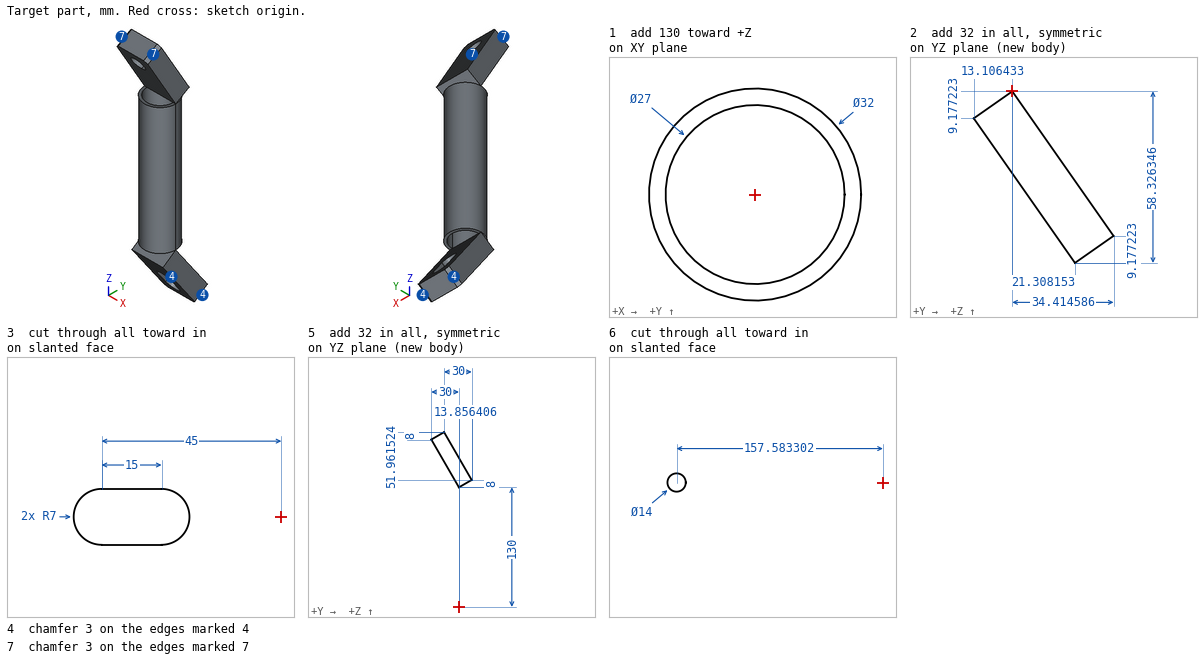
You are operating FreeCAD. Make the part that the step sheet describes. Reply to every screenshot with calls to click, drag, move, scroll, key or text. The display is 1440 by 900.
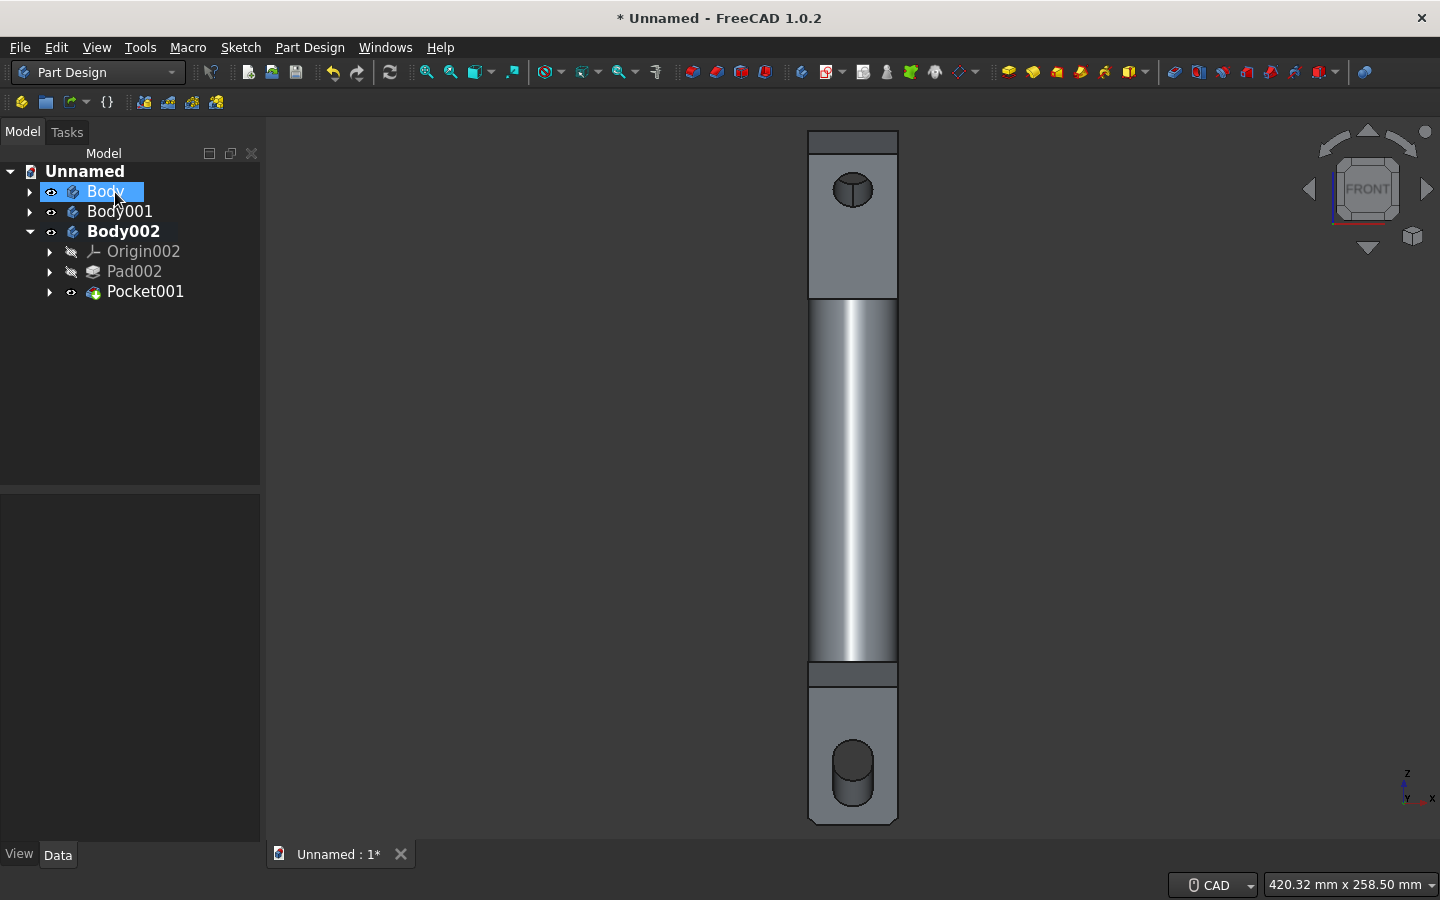
key(v)
key(f)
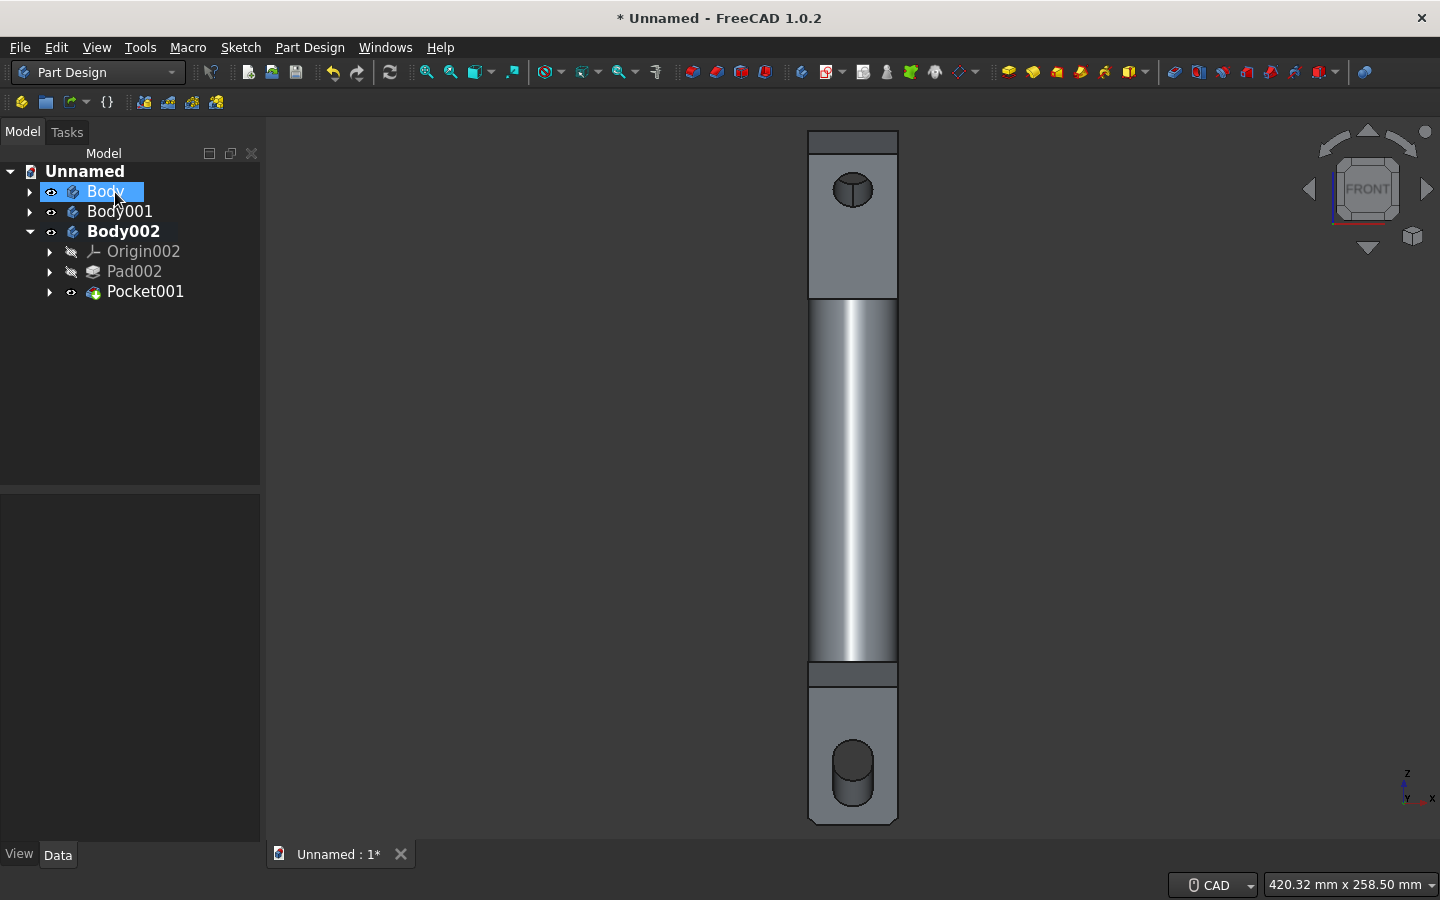
click(898, 146)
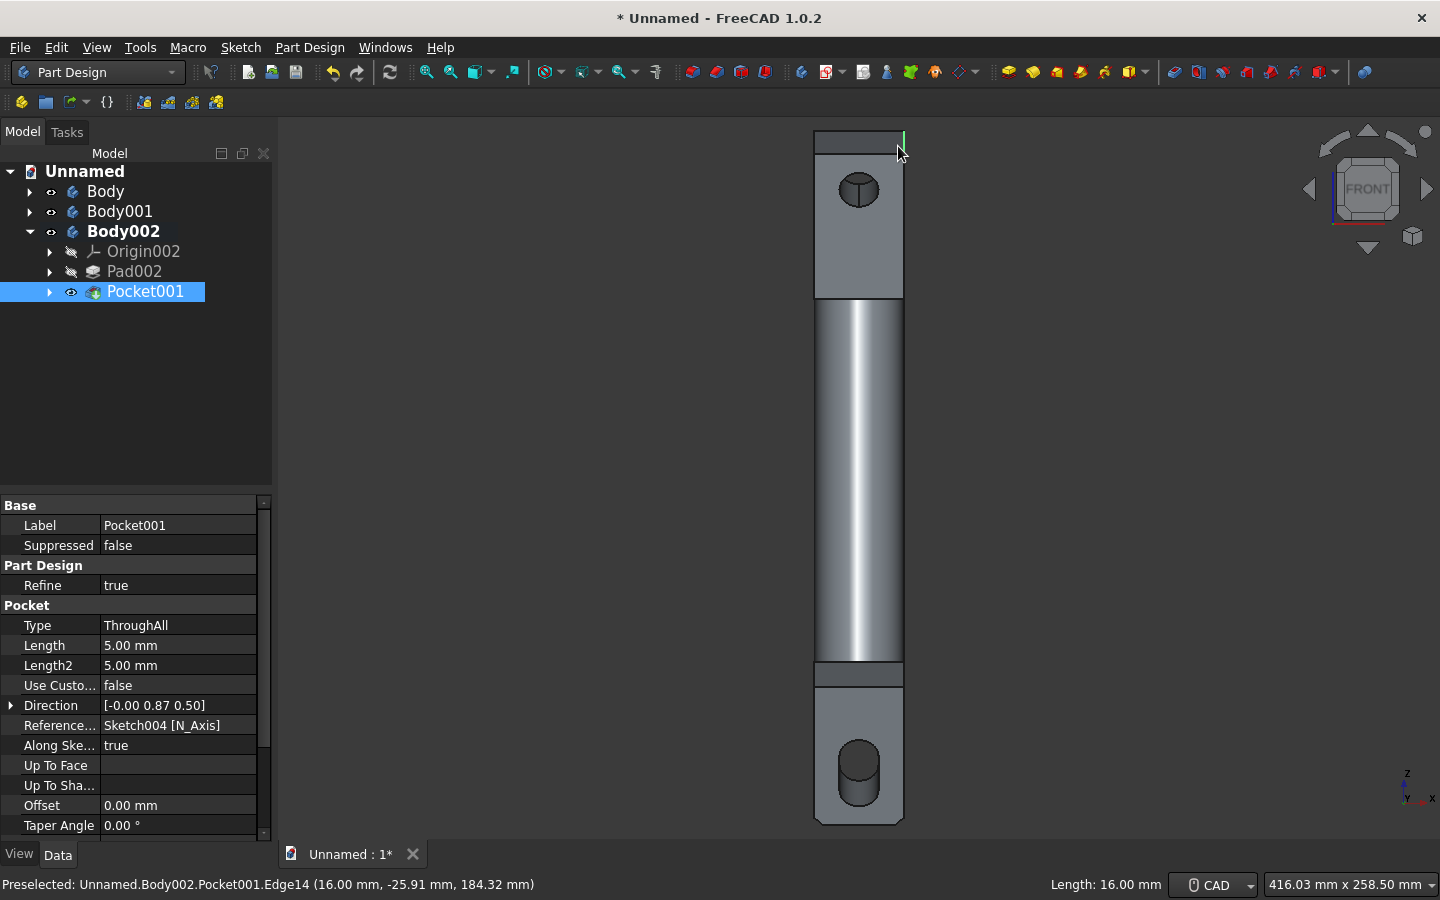
click(814, 146, ctrl)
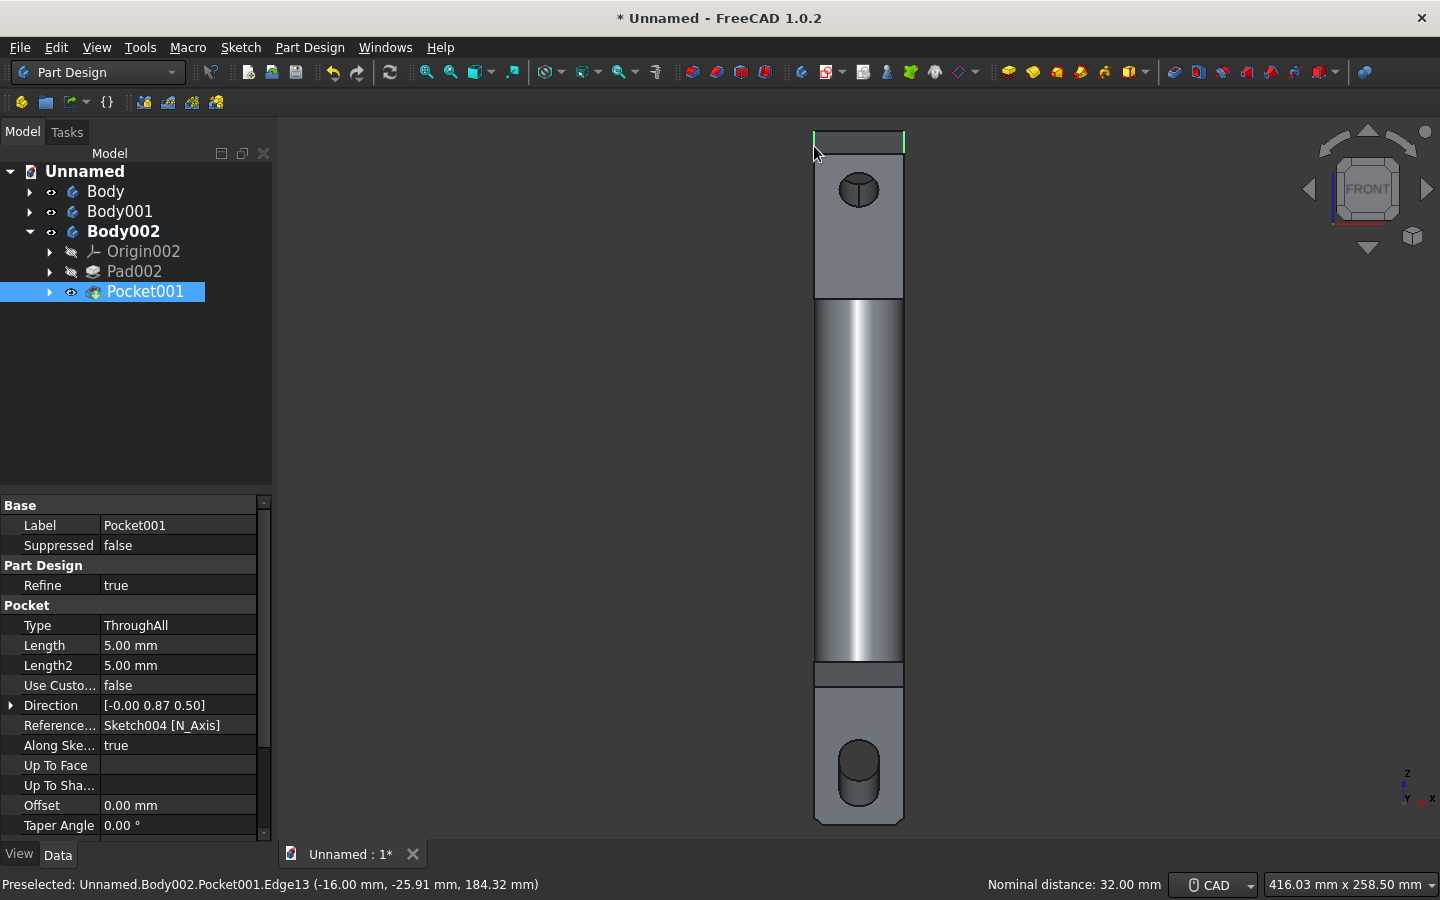
click(718, 72)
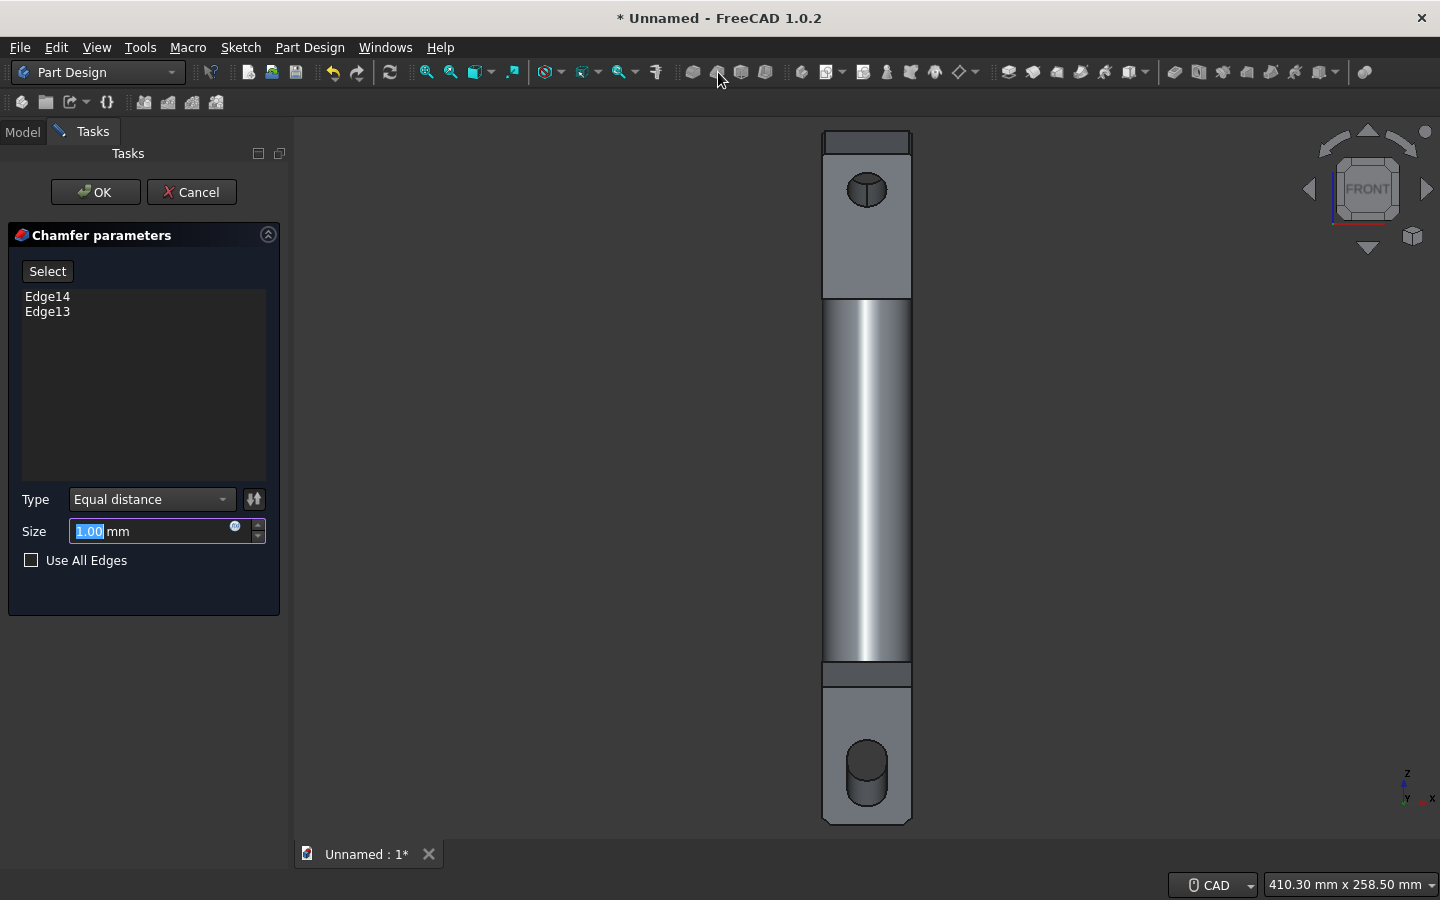
text(3)
key(Tab)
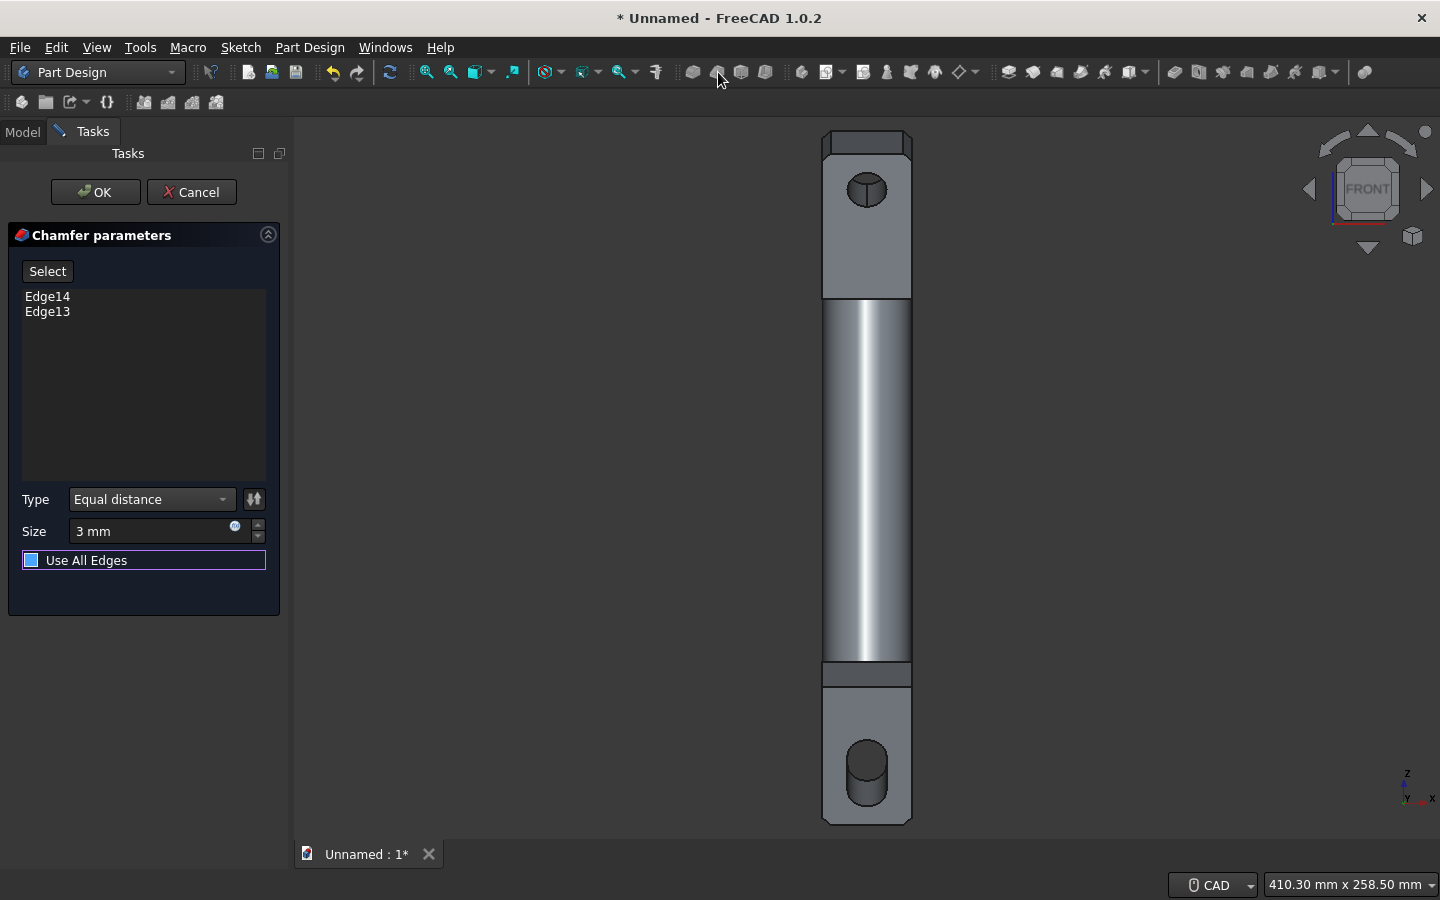
click(96, 192)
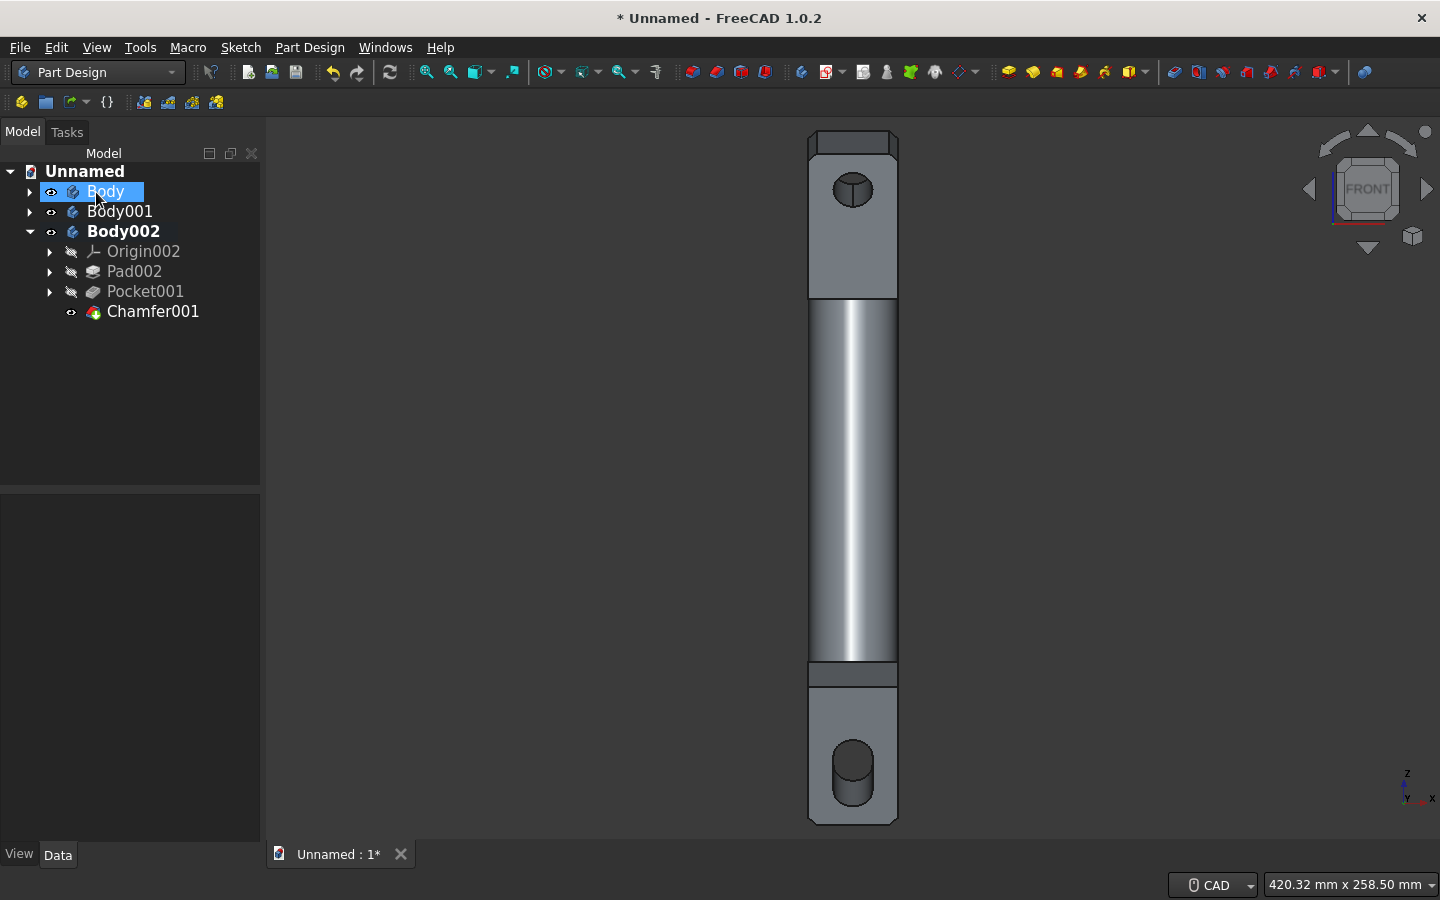
key(0)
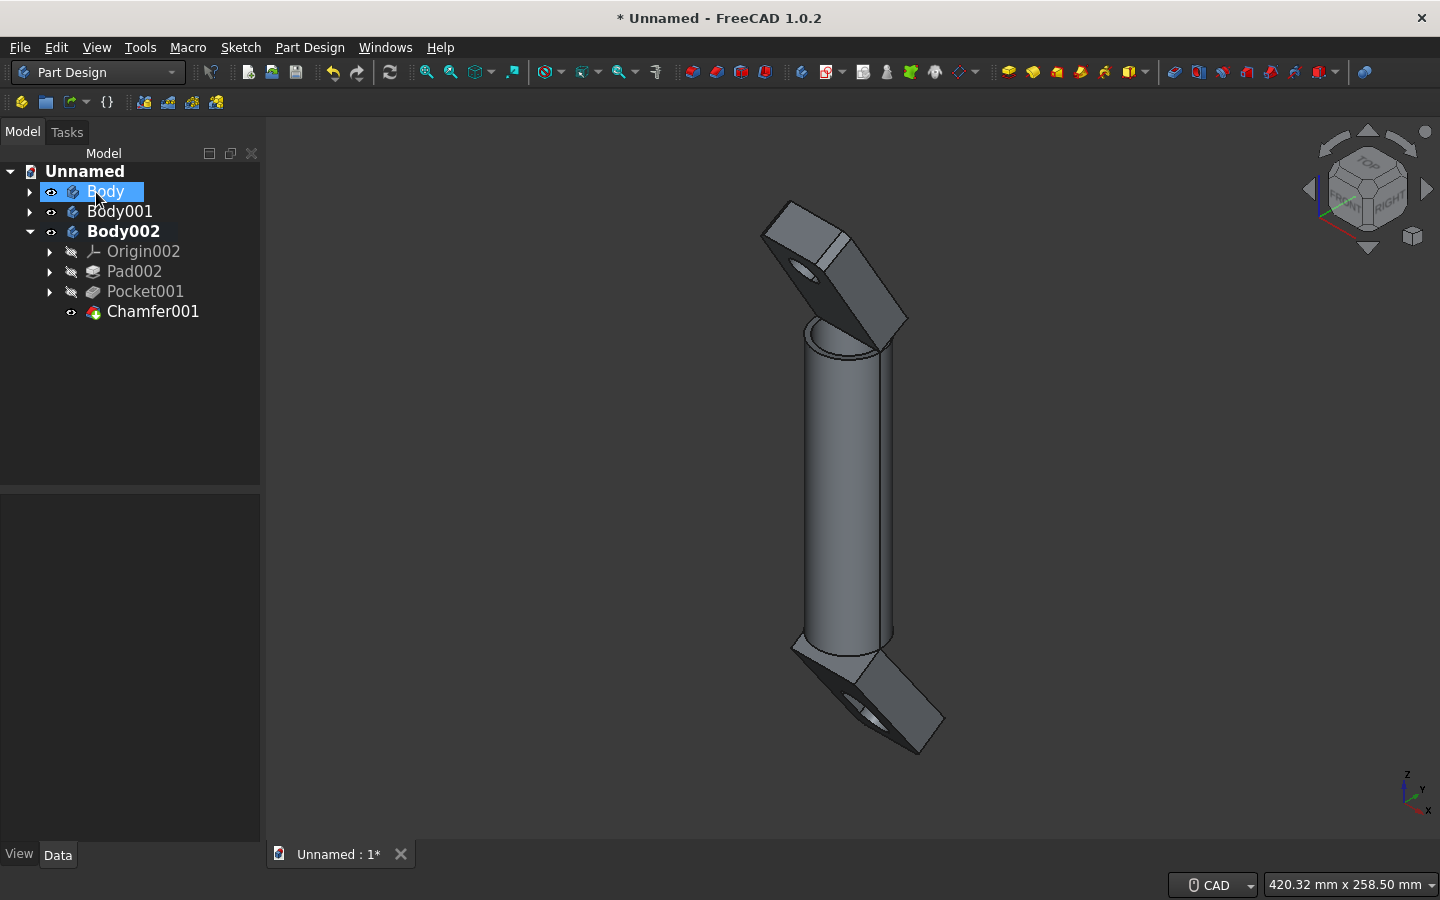
key(v)
key(f)